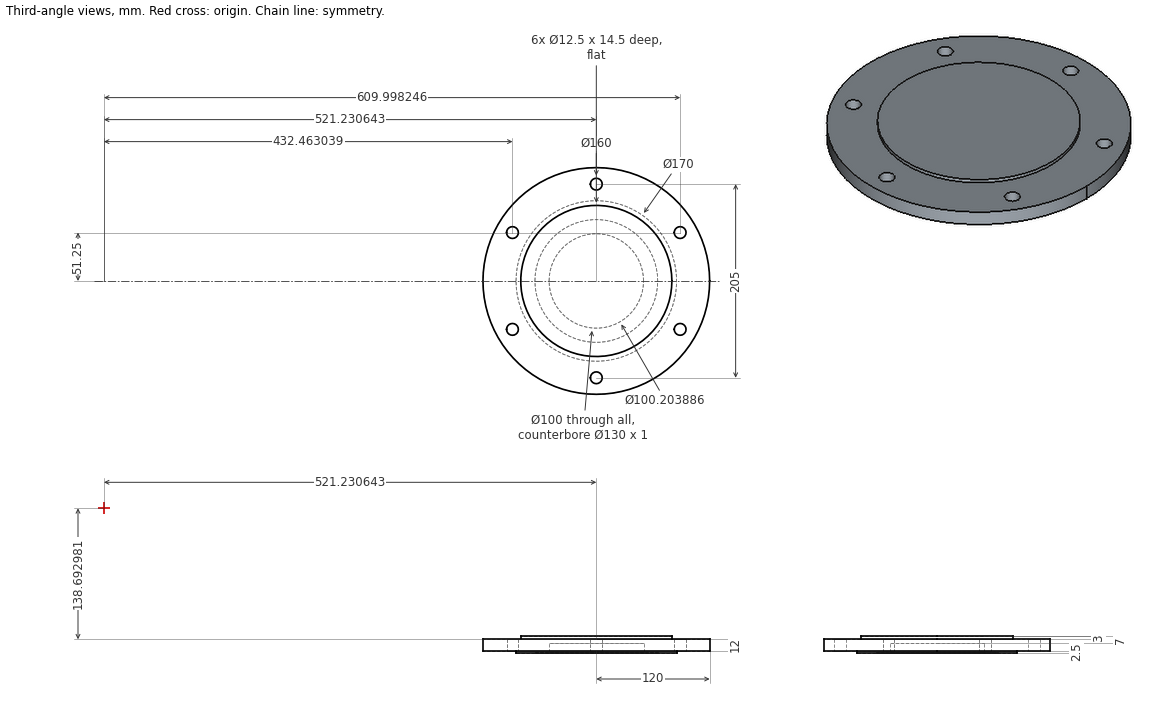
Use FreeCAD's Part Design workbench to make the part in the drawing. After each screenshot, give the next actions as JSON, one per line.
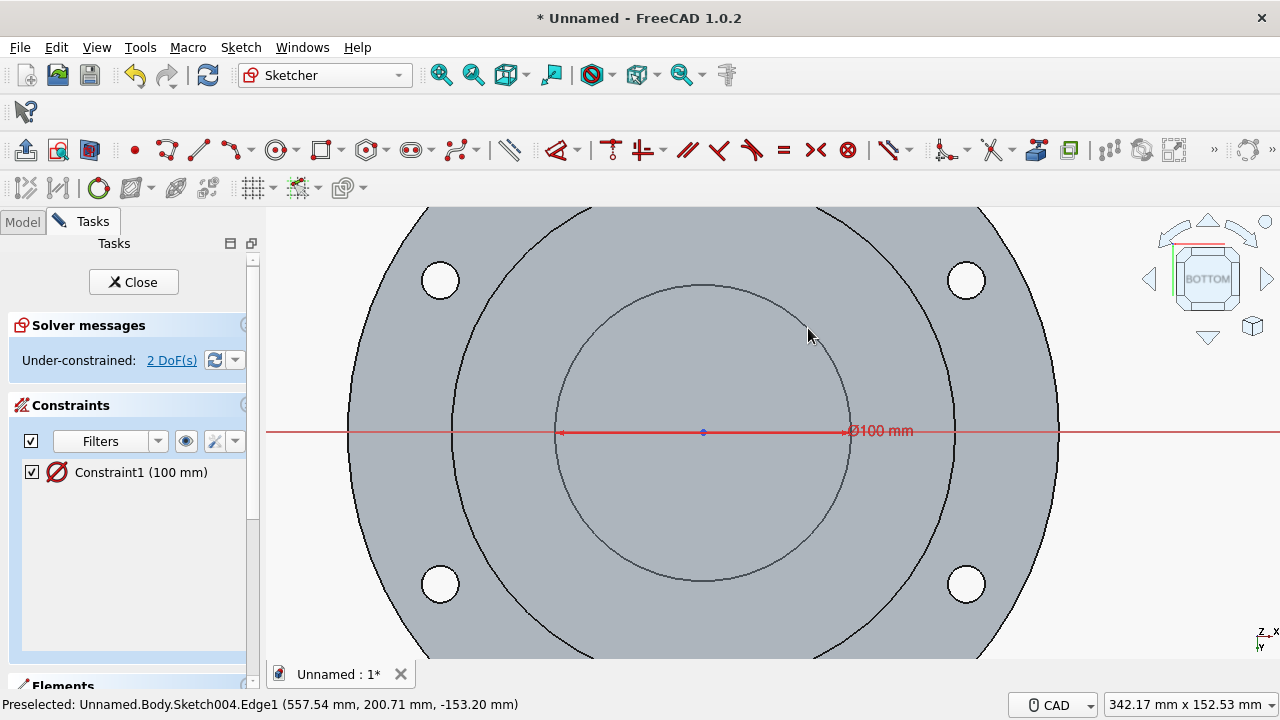
{"action": "left_click", "coordinate": [703, 433]}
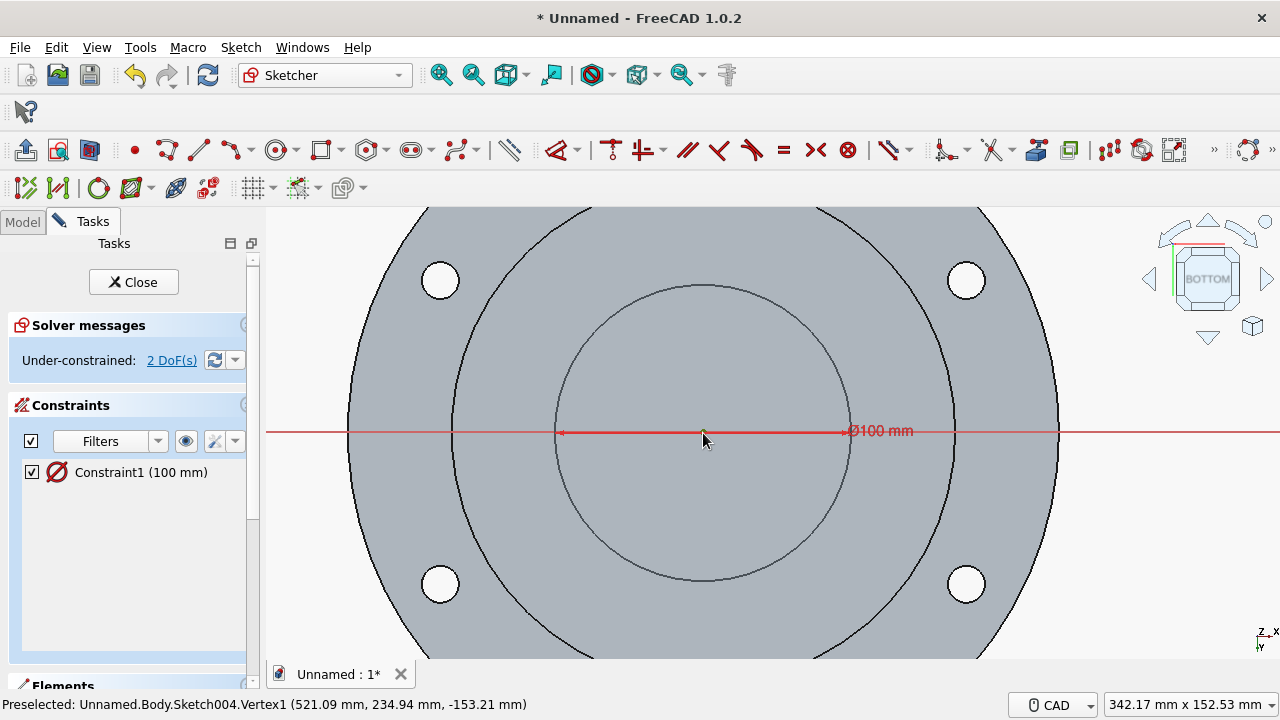
{"action": "left_click", "coordinate": [353, 432]}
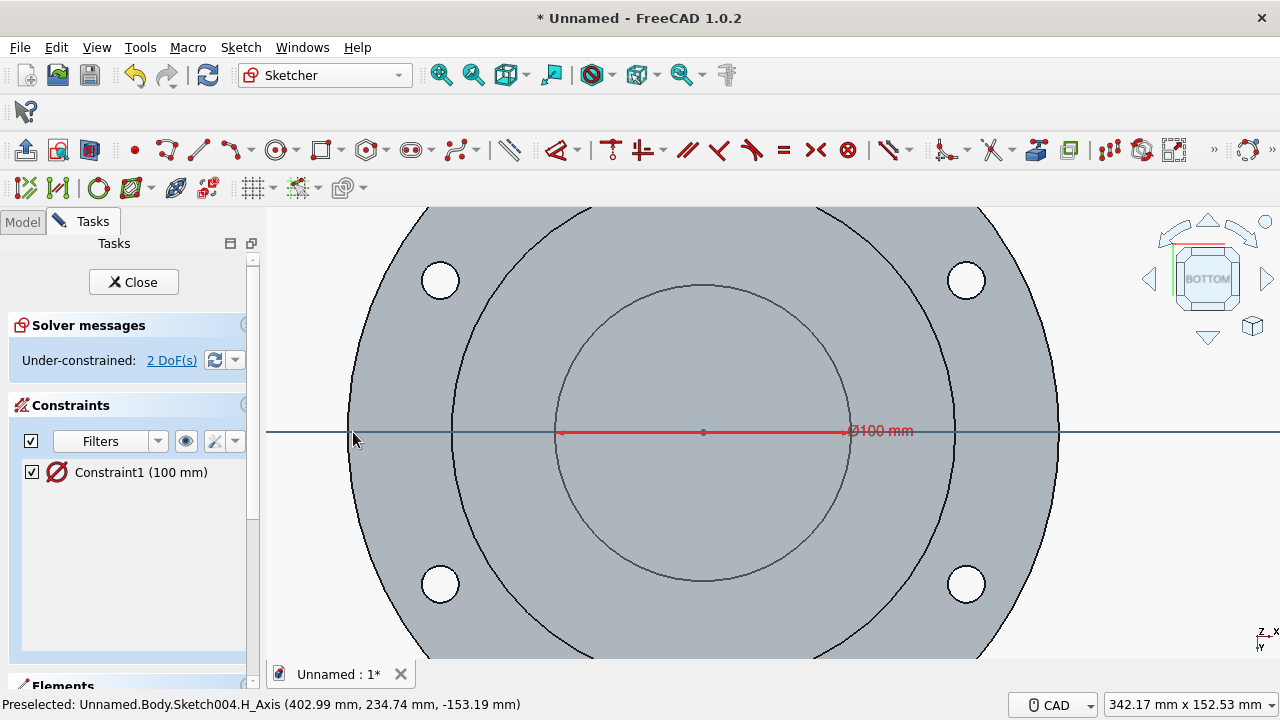
{"action": "left_click", "coordinate": [612, 150]}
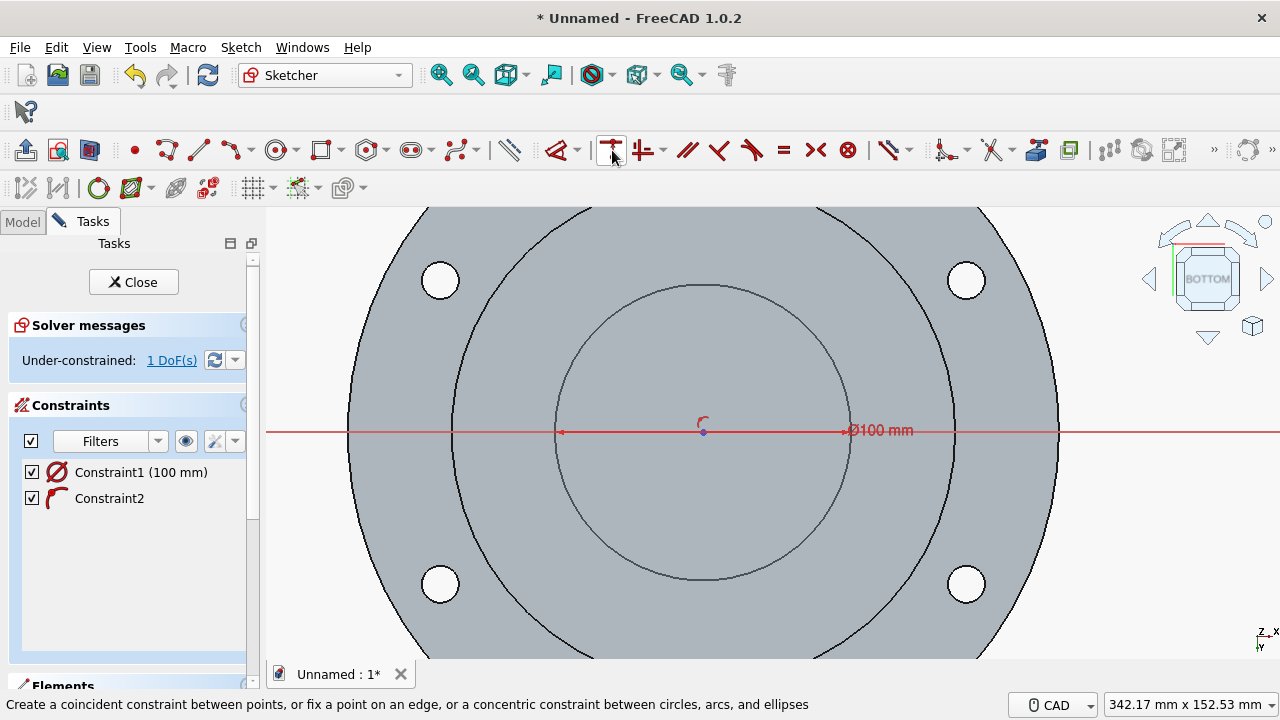
{"action": "key", "text": "d"}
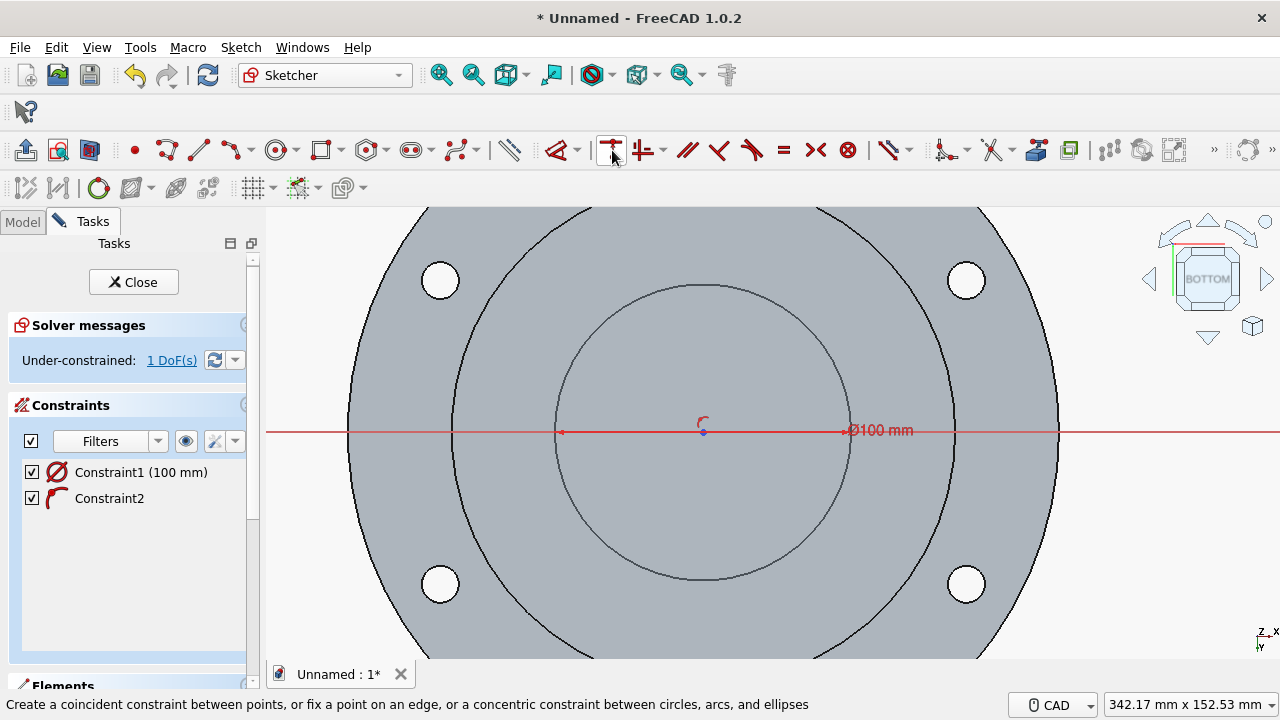
{"action": "left_click", "coordinate": [703, 432]}
{"action": "left_click", "coordinate": [499, 466]}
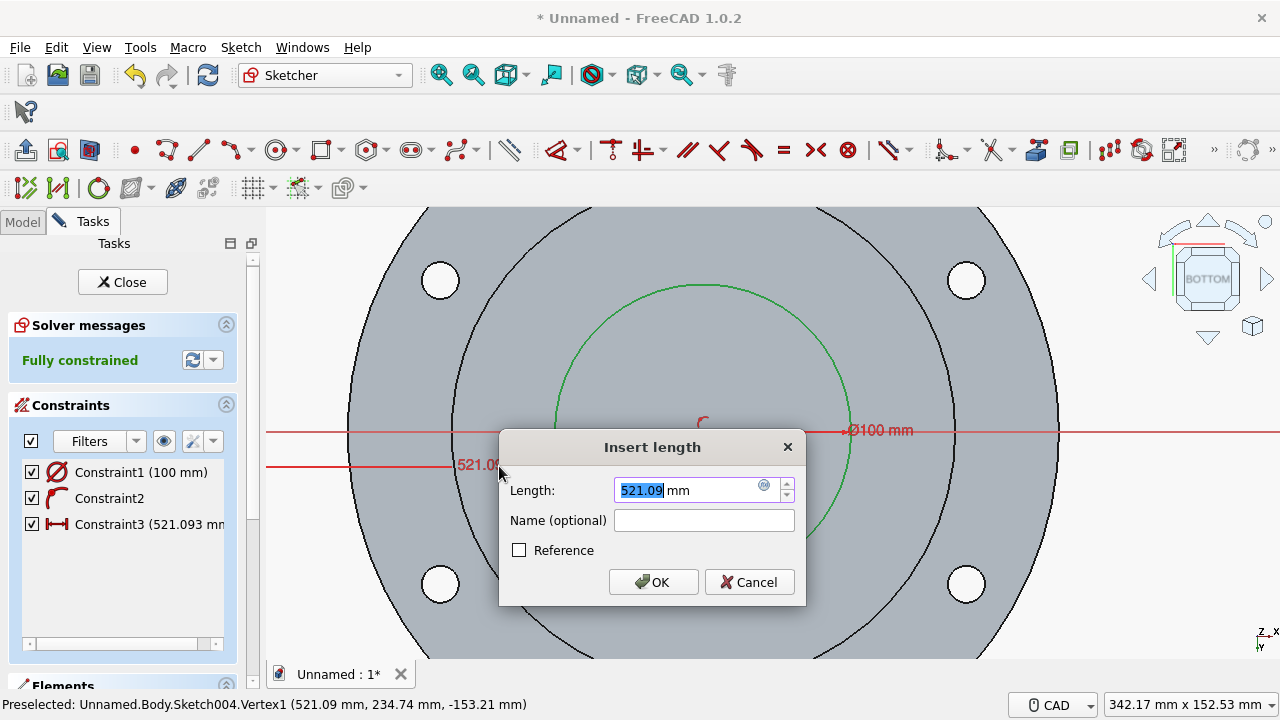
{"action": "type", "text": "521.230643"}
{"action": "key", "text": "Return"}
{"action": "key", "text": "Escape"}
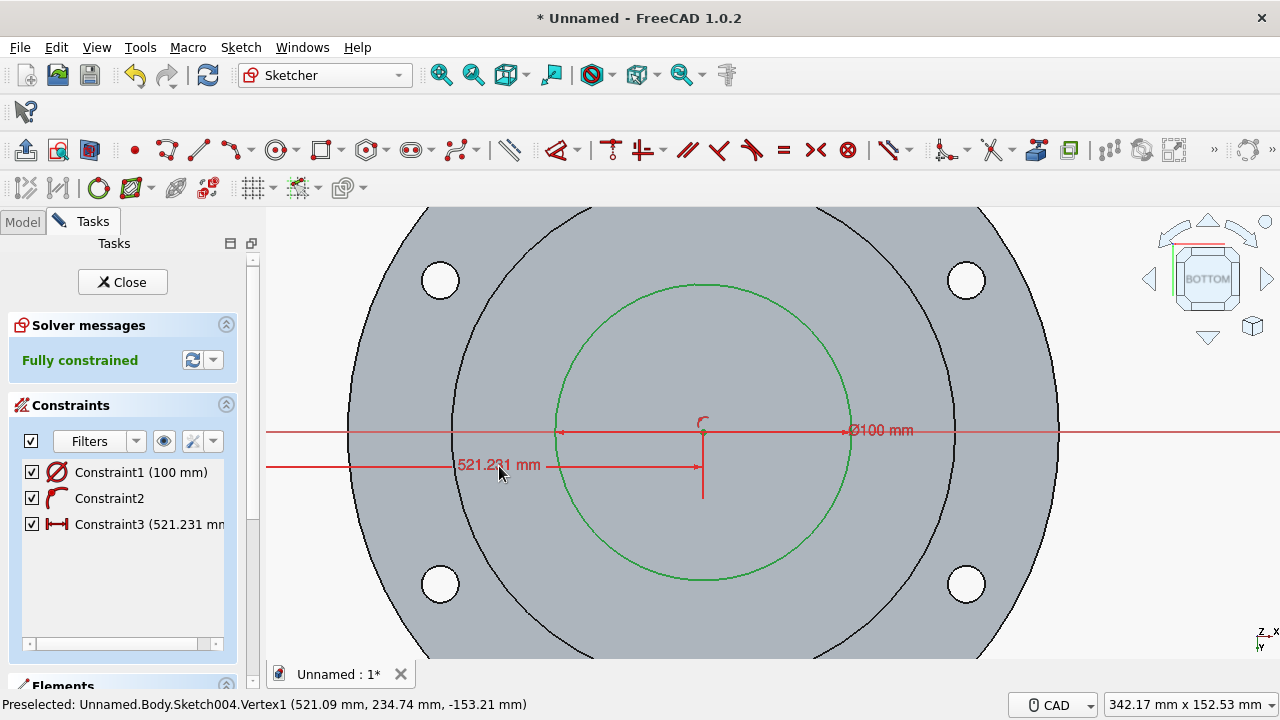
{"action": "left_click", "coordinate": [123, 282]}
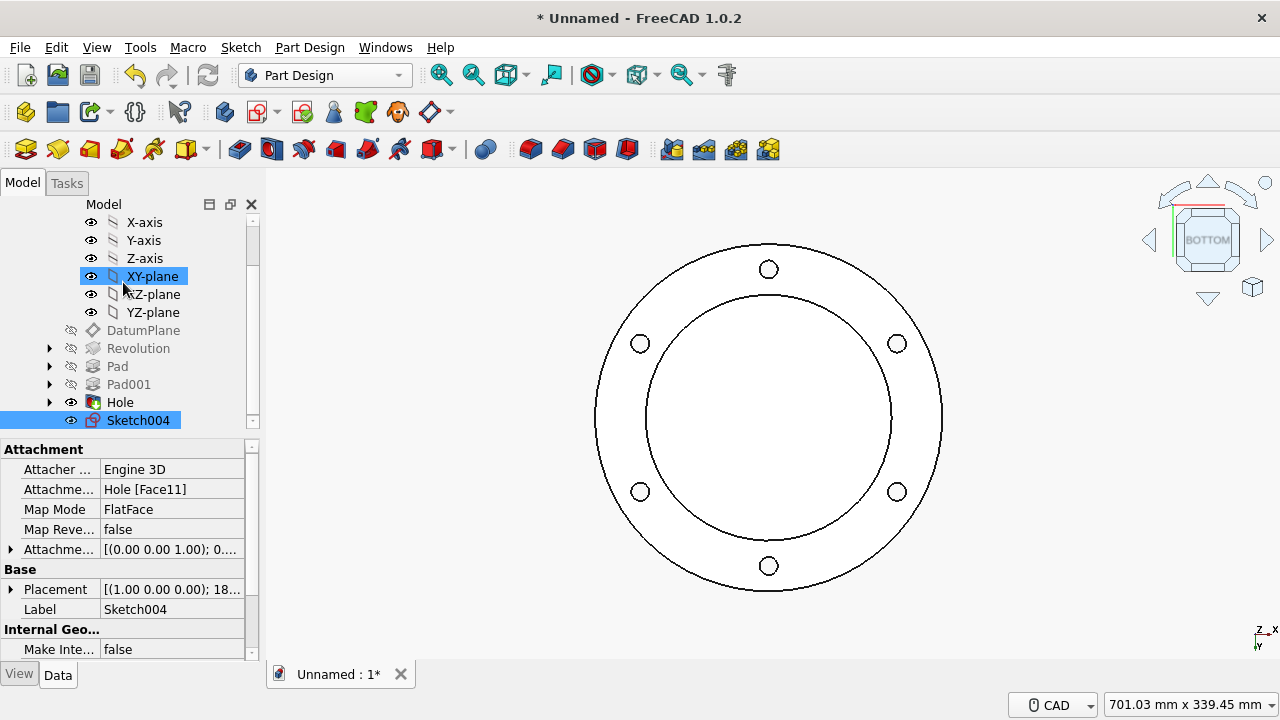
{"action": "left_click", "coordinate": [272, 150]}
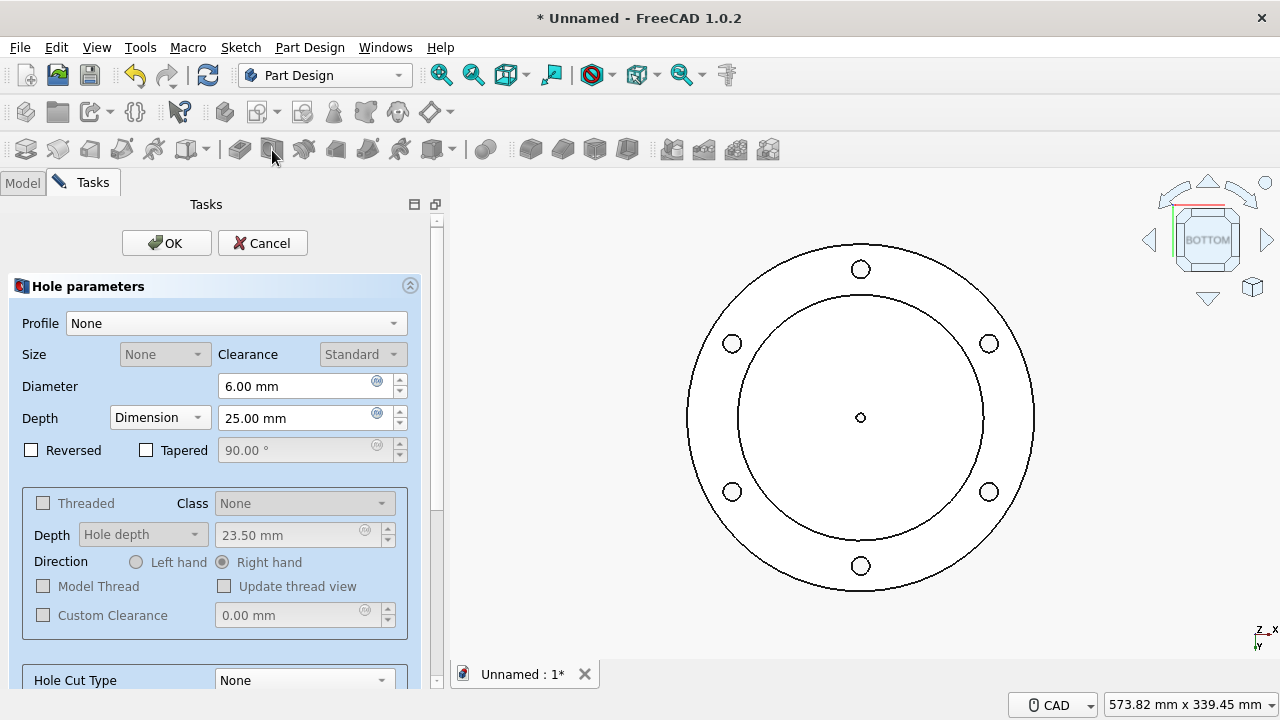
{"action": "triple_click", "coordinate": [305, 386]}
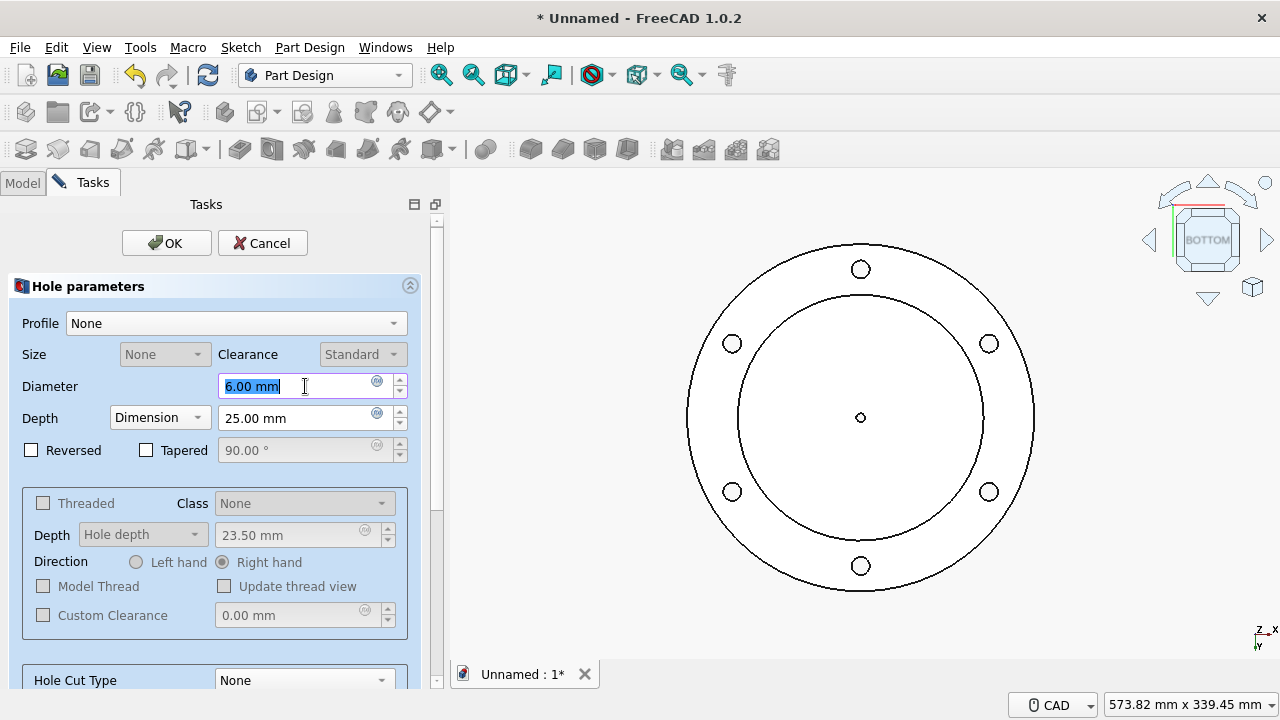
{"action": "type", "text": "100"}
{"action": "key", "text": "Tab"}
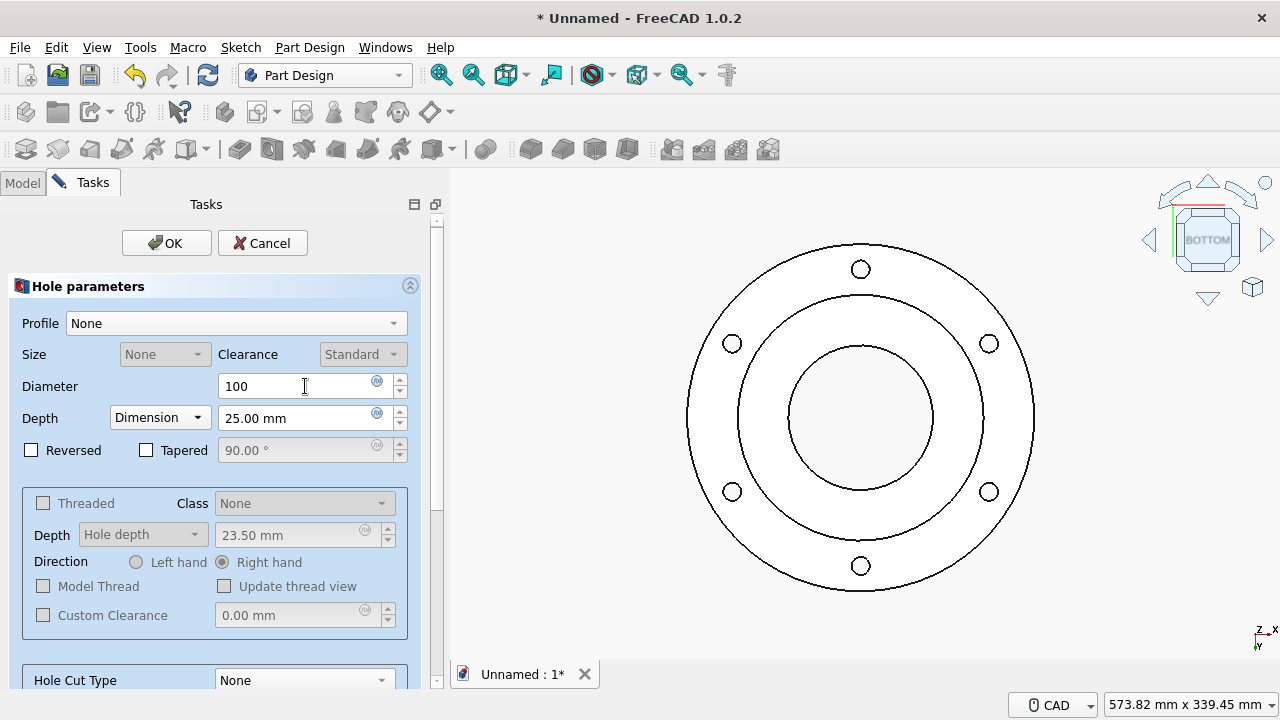
{"action": "left_click", "coordinate": [161, 418]}